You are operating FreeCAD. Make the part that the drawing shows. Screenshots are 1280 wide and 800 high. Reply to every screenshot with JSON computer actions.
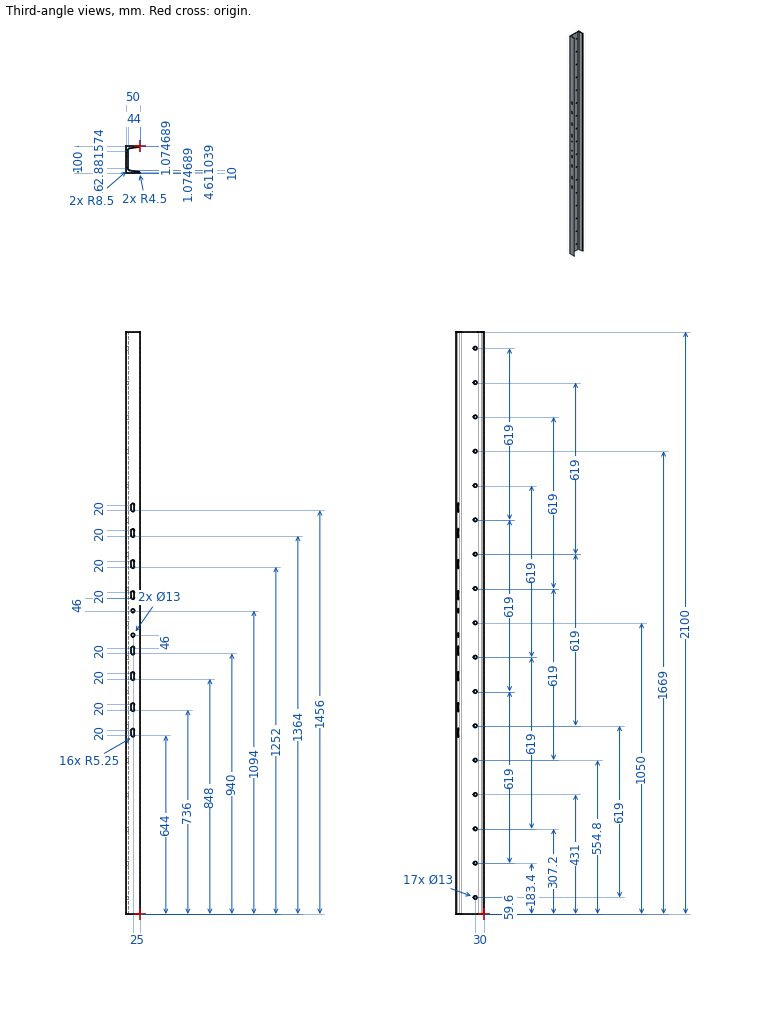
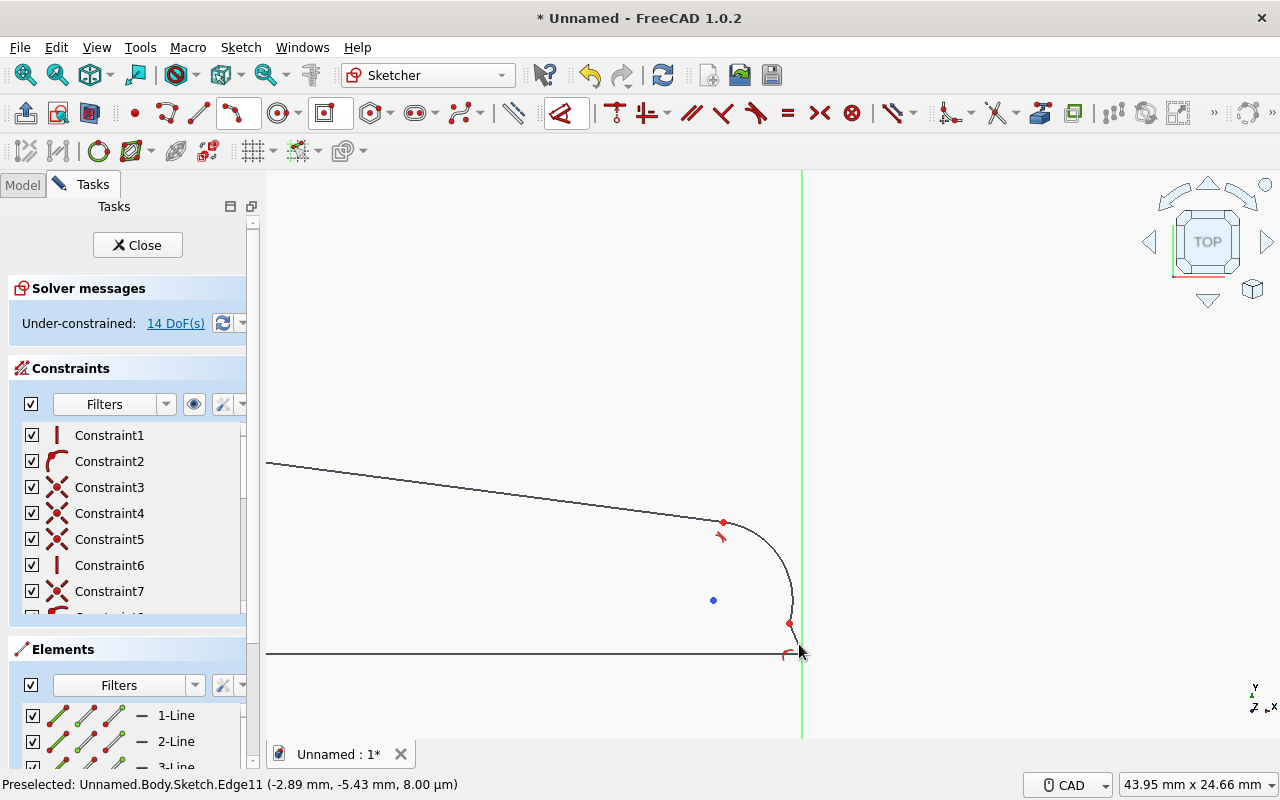
{"action": "left_click", "coordinate": [796, 639]}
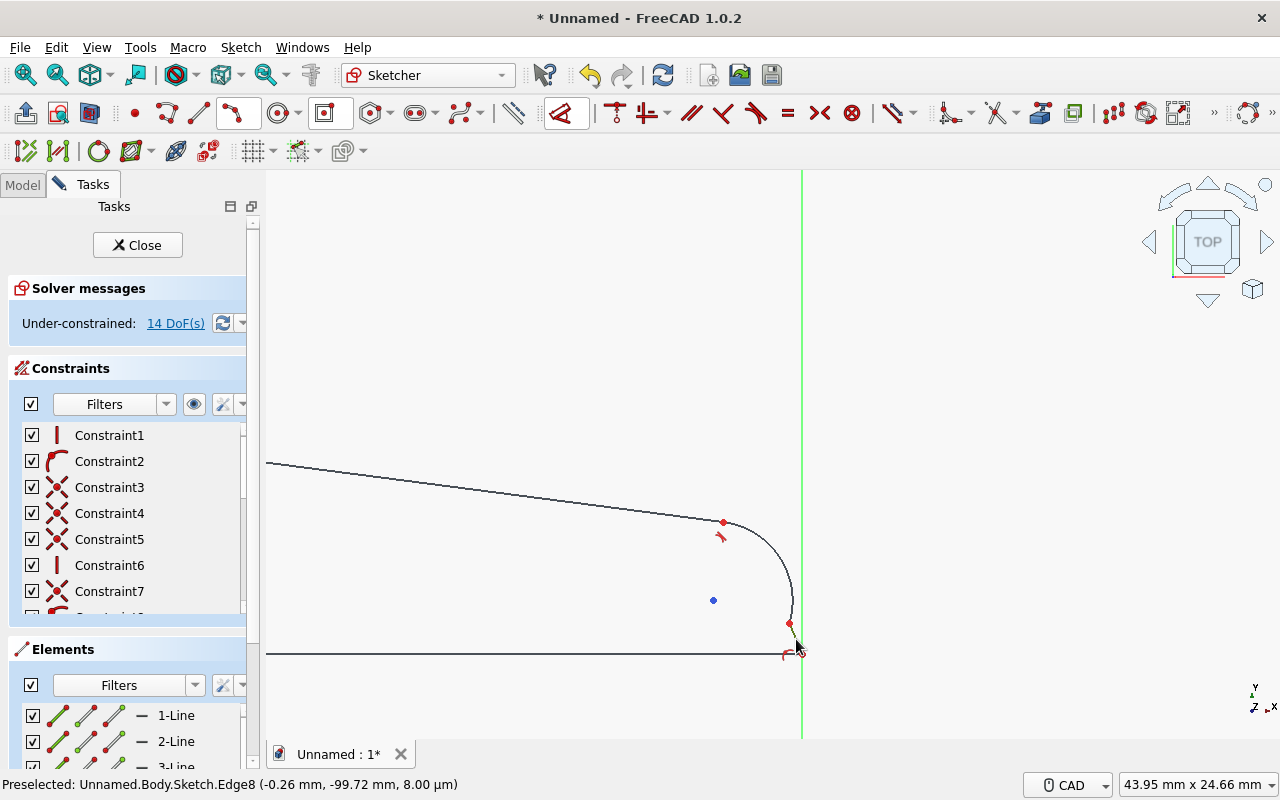
{"action": "left_click", "coordinate": [791, 583]}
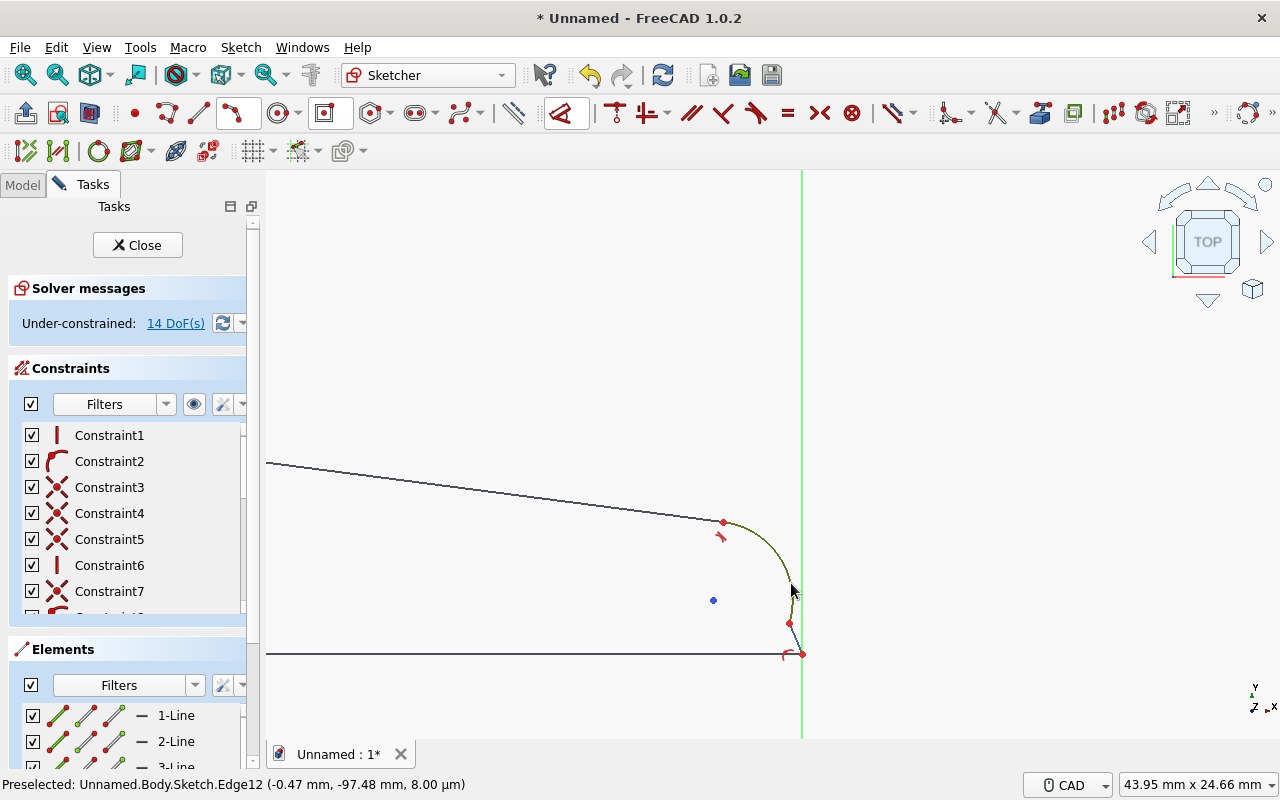
{"action": "left_click", "coordinate": [756, 114]}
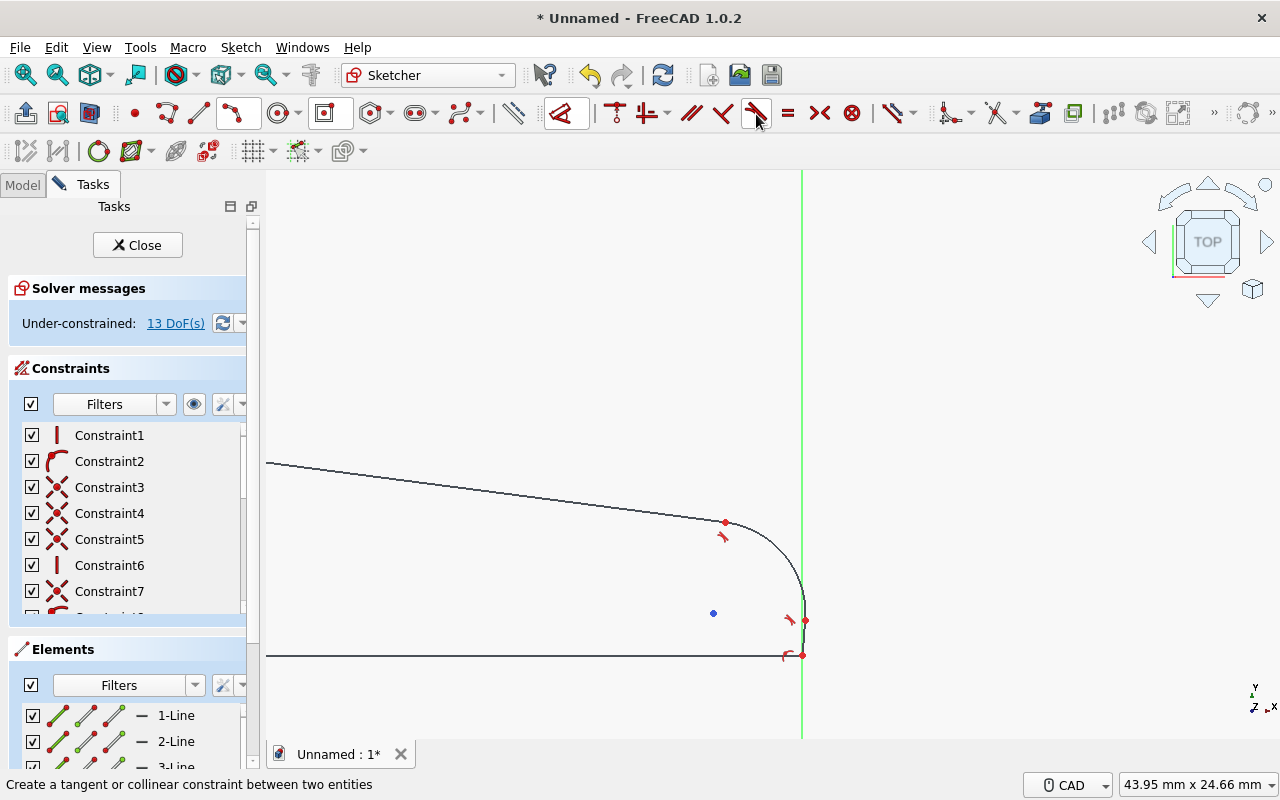
{"action": "scroll", "coordinate": [799, 645], "scroll_direction": "down", "scroll_amount": 9}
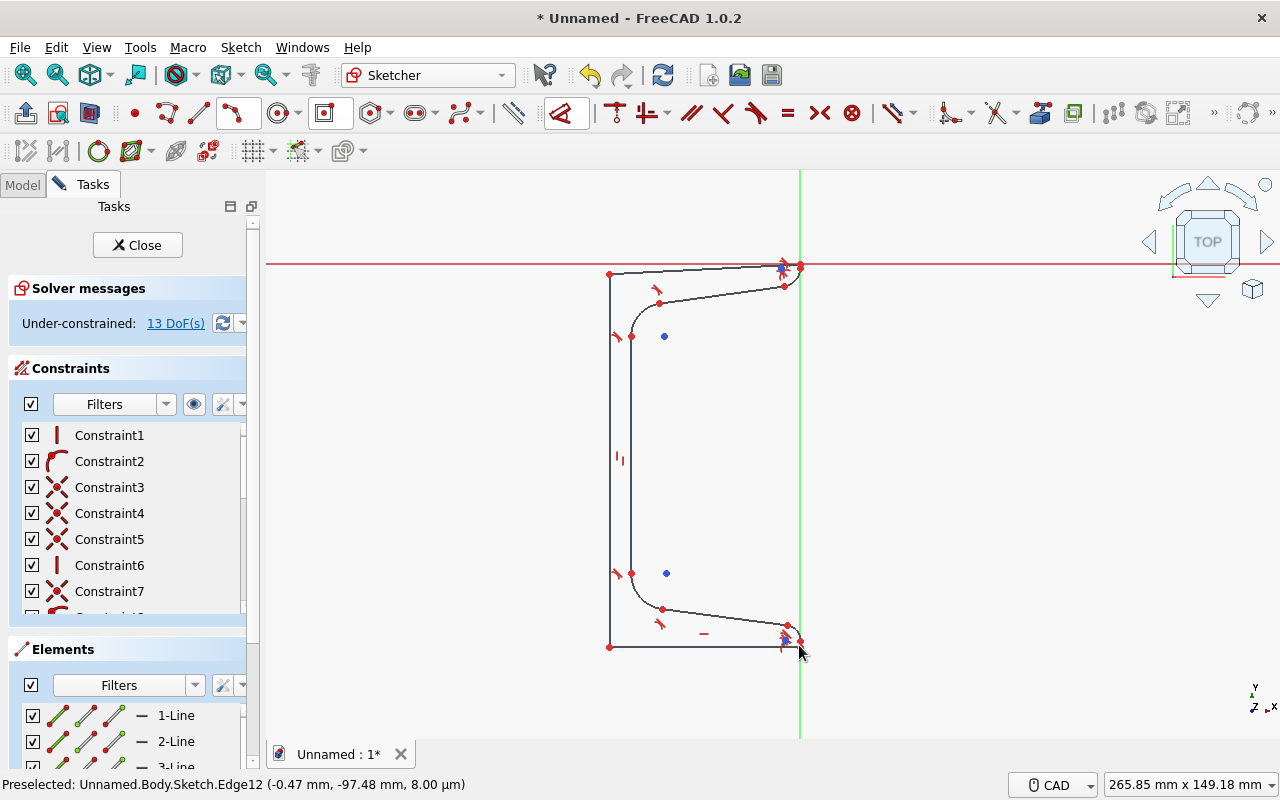
{"action": "scroll", "coordinate": [743, 267], "scroll_direction": "up", "scroll_amount": 8}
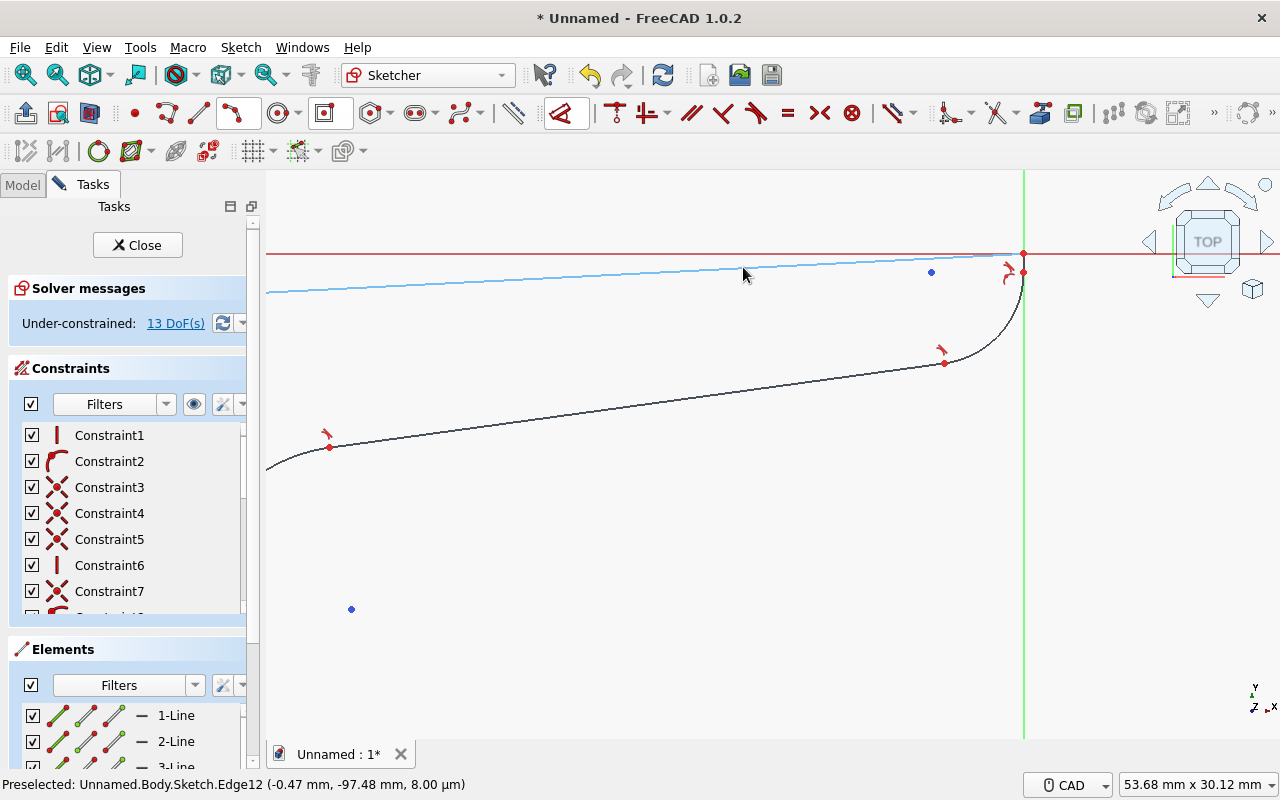
{"action": "left_click", "coordinate": [741, 268]}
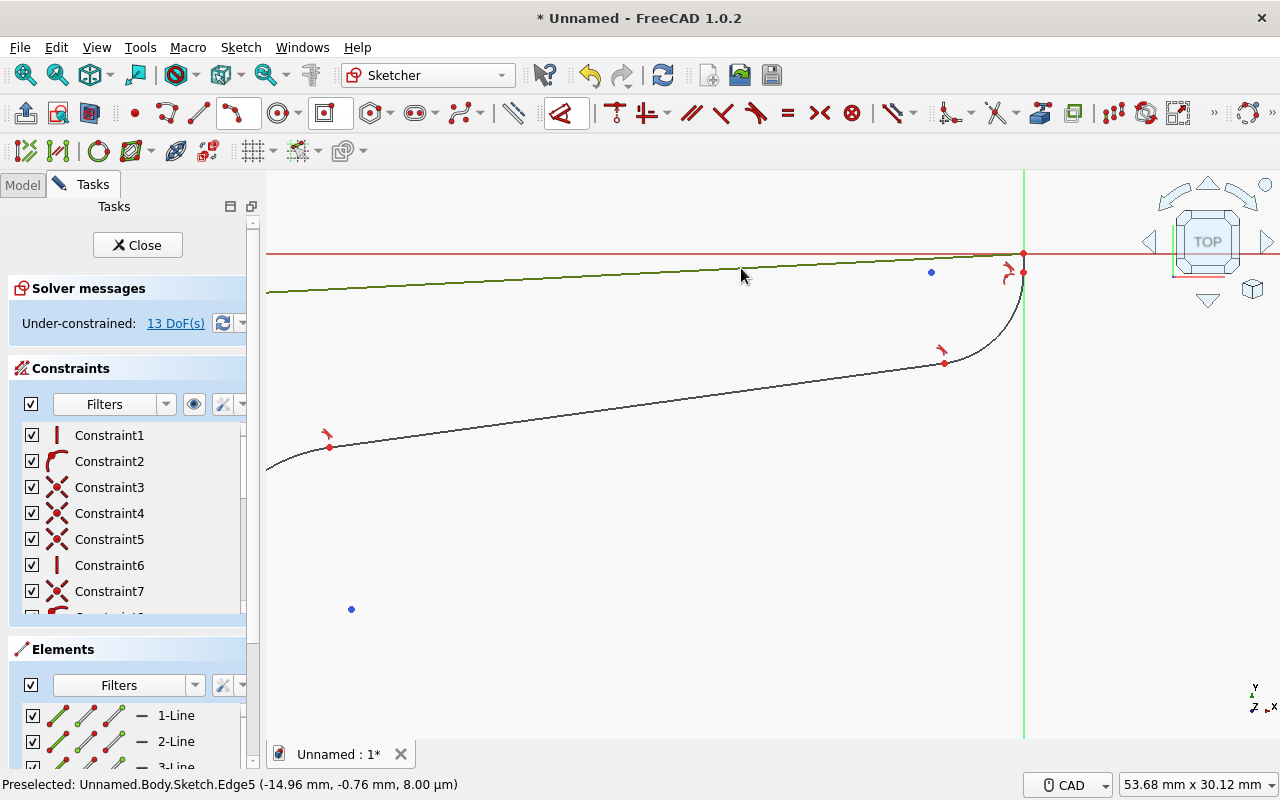
{"action": "left_click", "coordinate": [670, 114]}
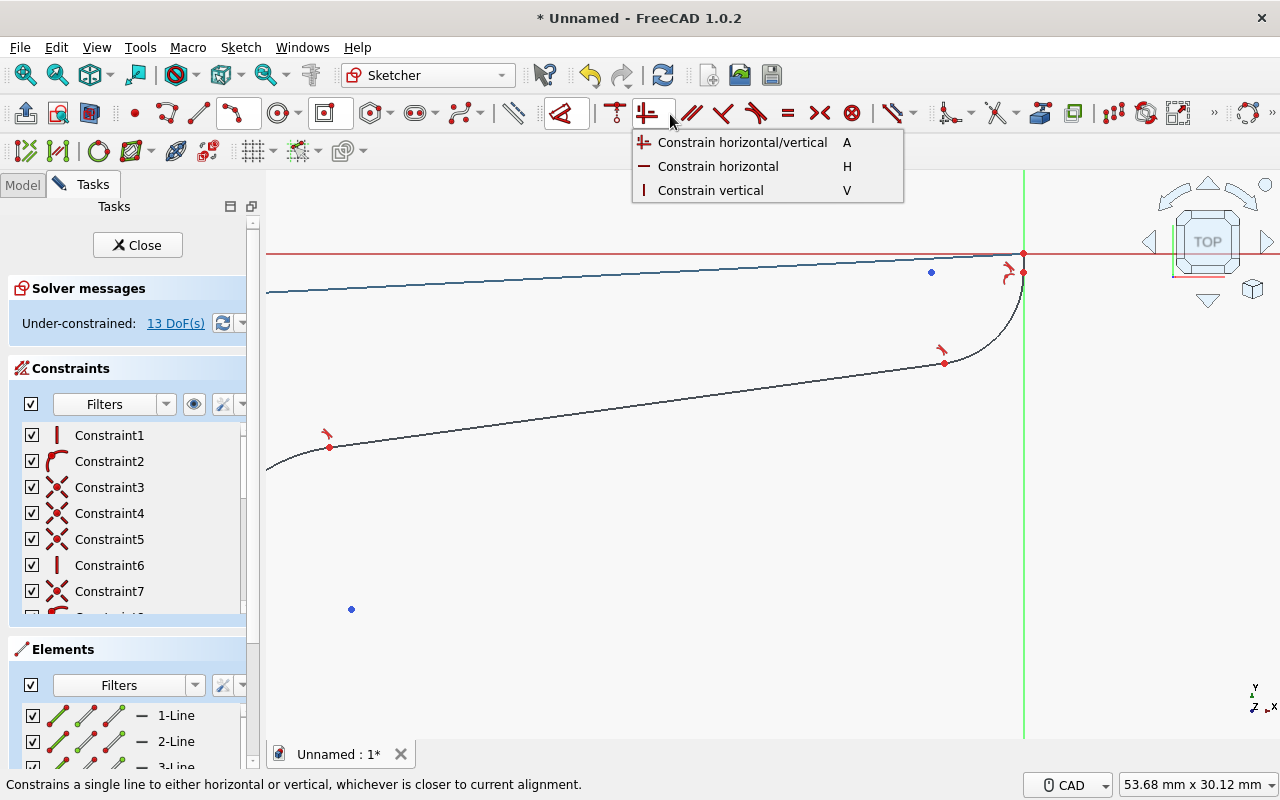
{"action": "left_click", "coordinate": [768, 166]}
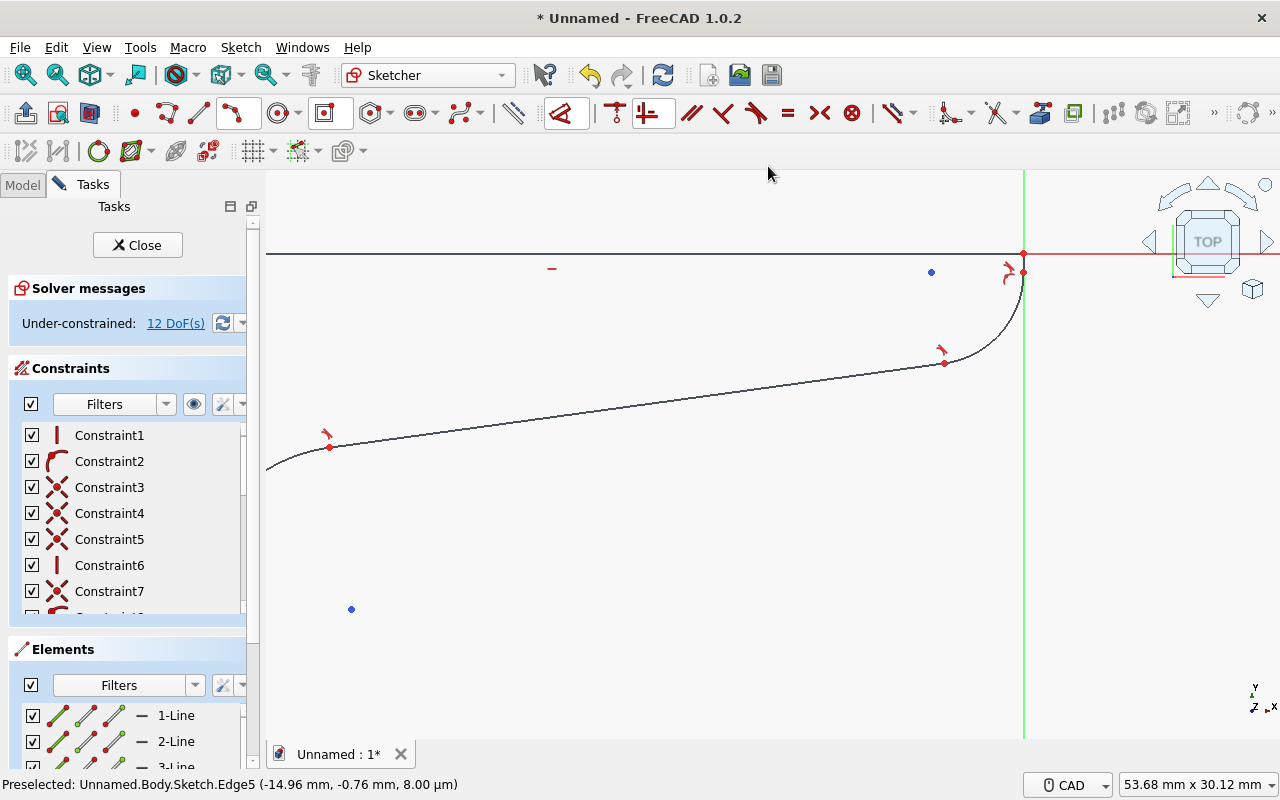
{"action": "scroll", "coordinate": [743, 266], "scroll_direction": "down", "scroll_amount": 8}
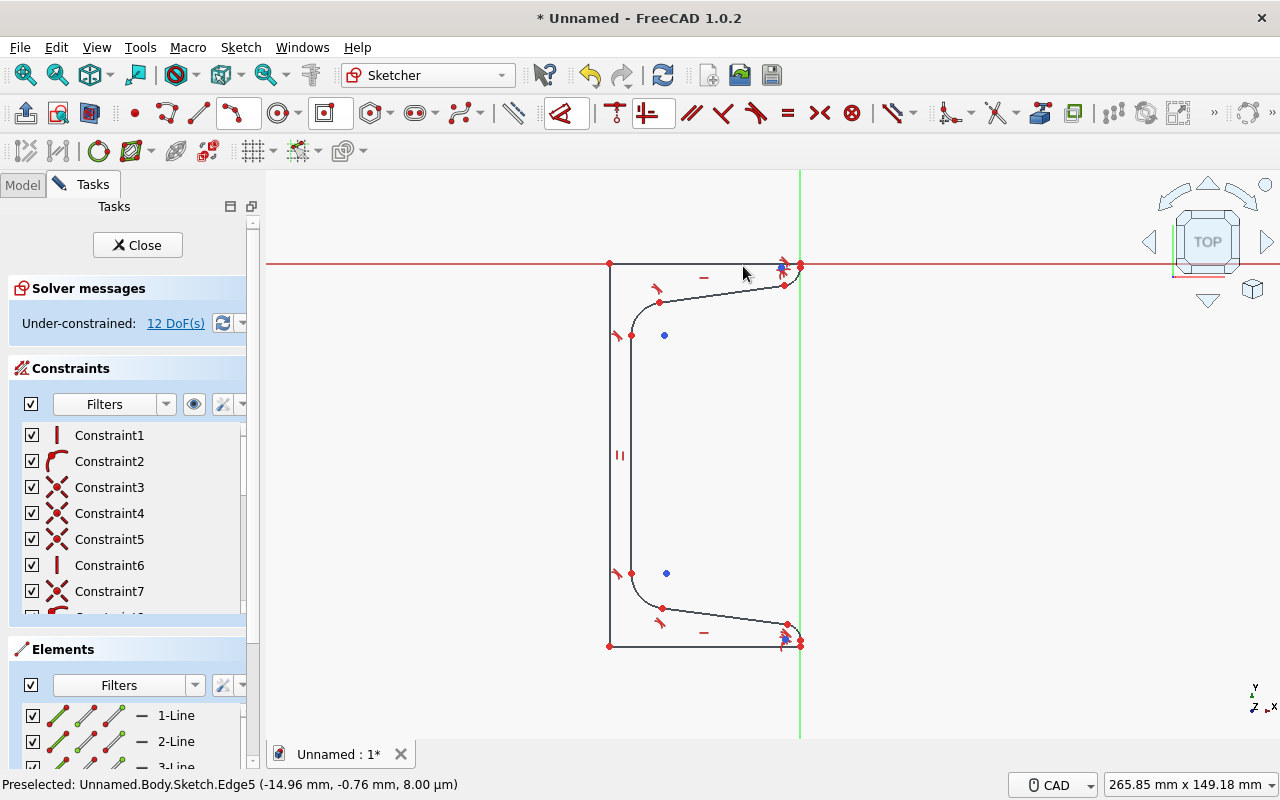
{"action": "scroll", "coordinate": [800, 644], "scroll_direction": "up", "scroll_amount": 9}